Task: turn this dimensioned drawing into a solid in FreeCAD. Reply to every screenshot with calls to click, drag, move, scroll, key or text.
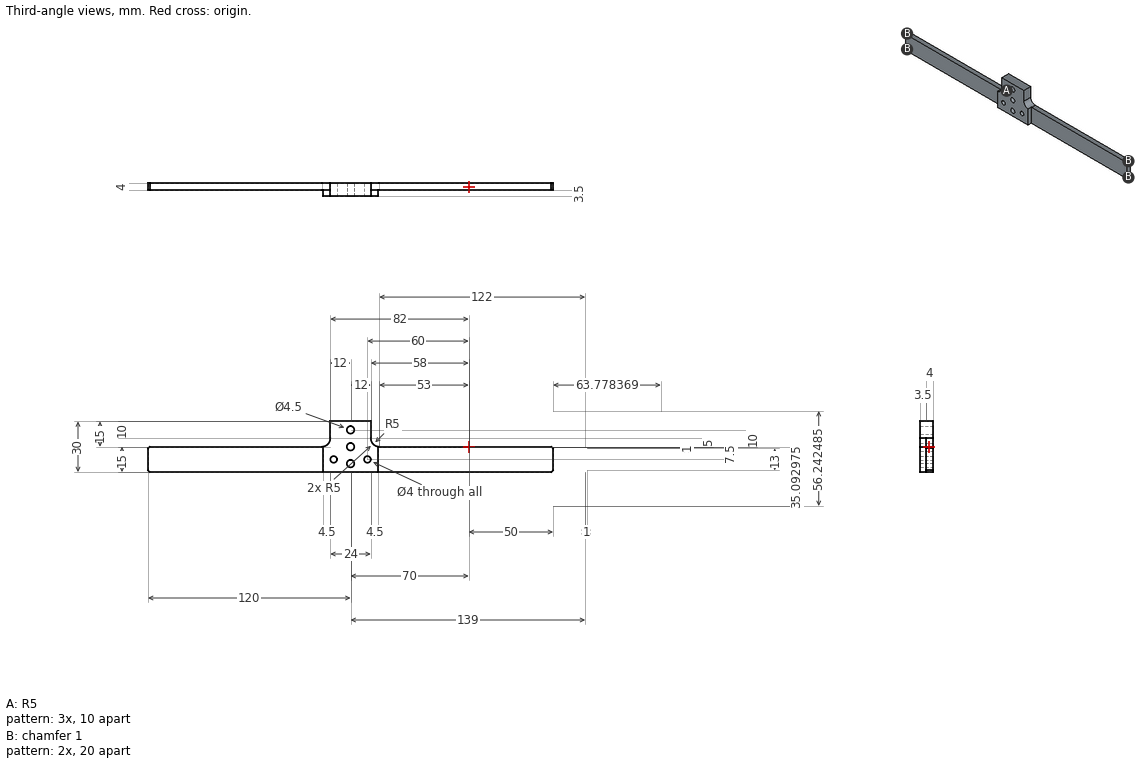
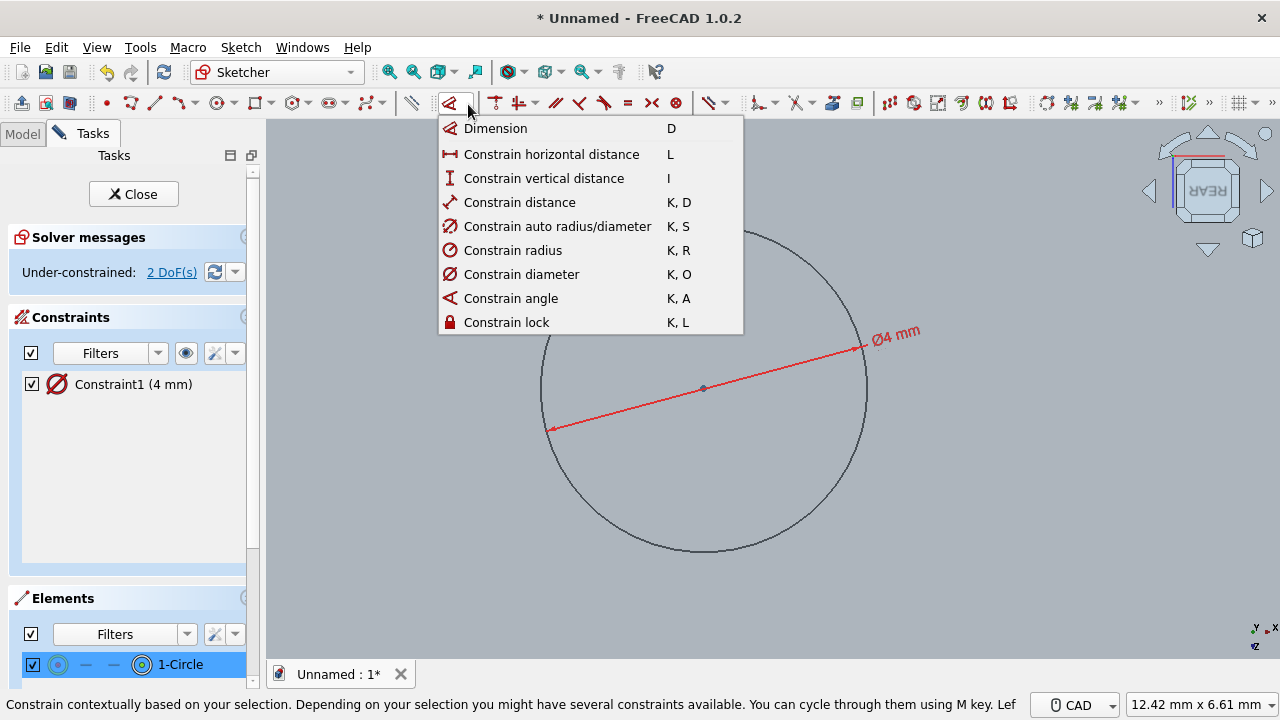
click(591, 154)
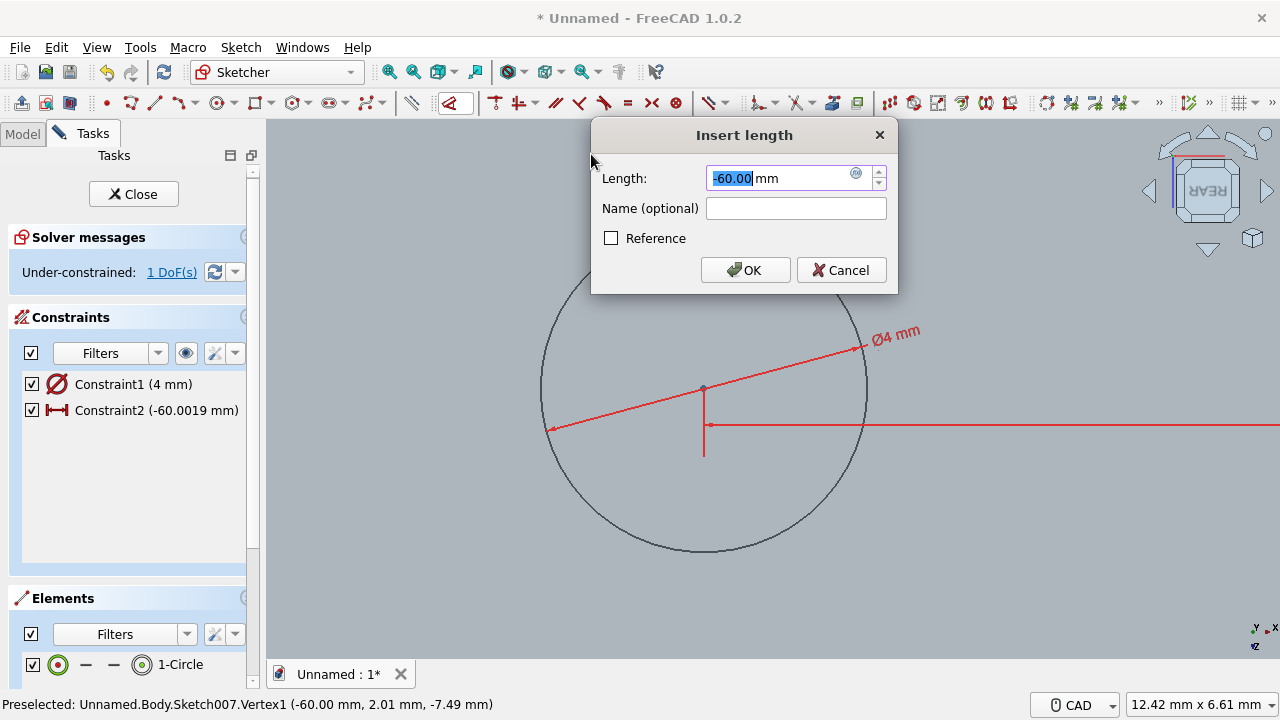
text(-60)
key(Return)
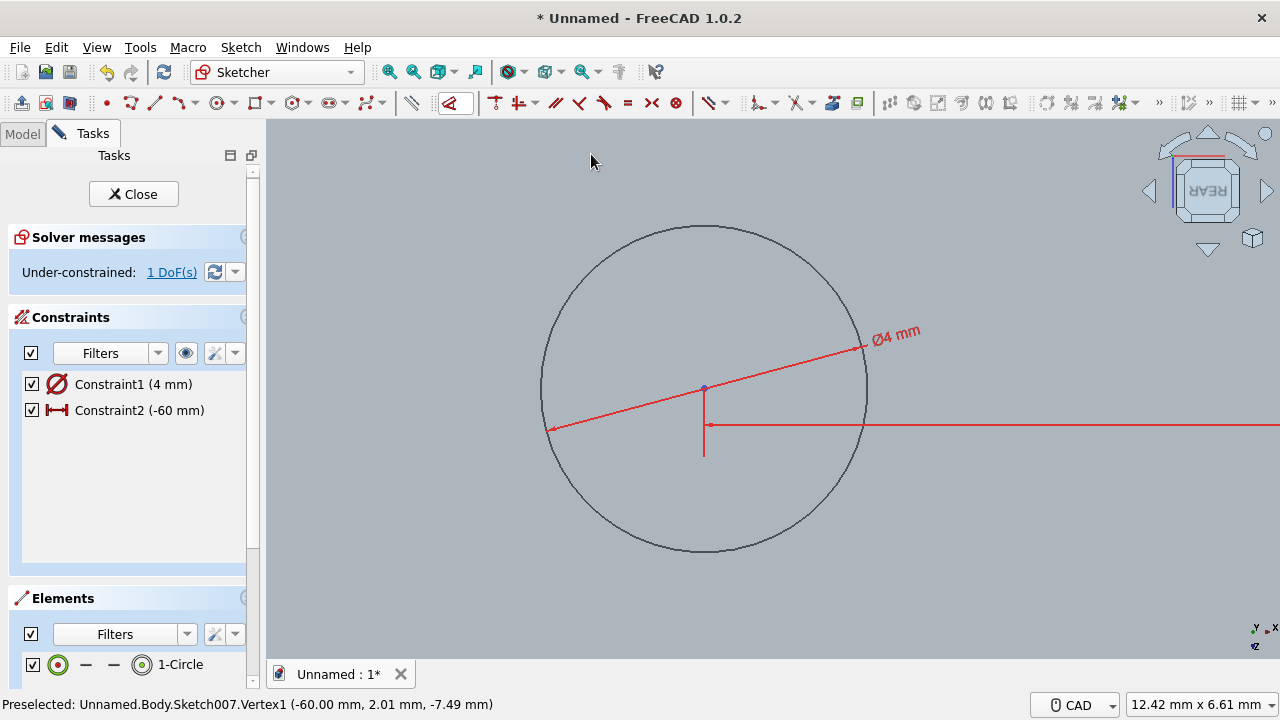
click(704, 389)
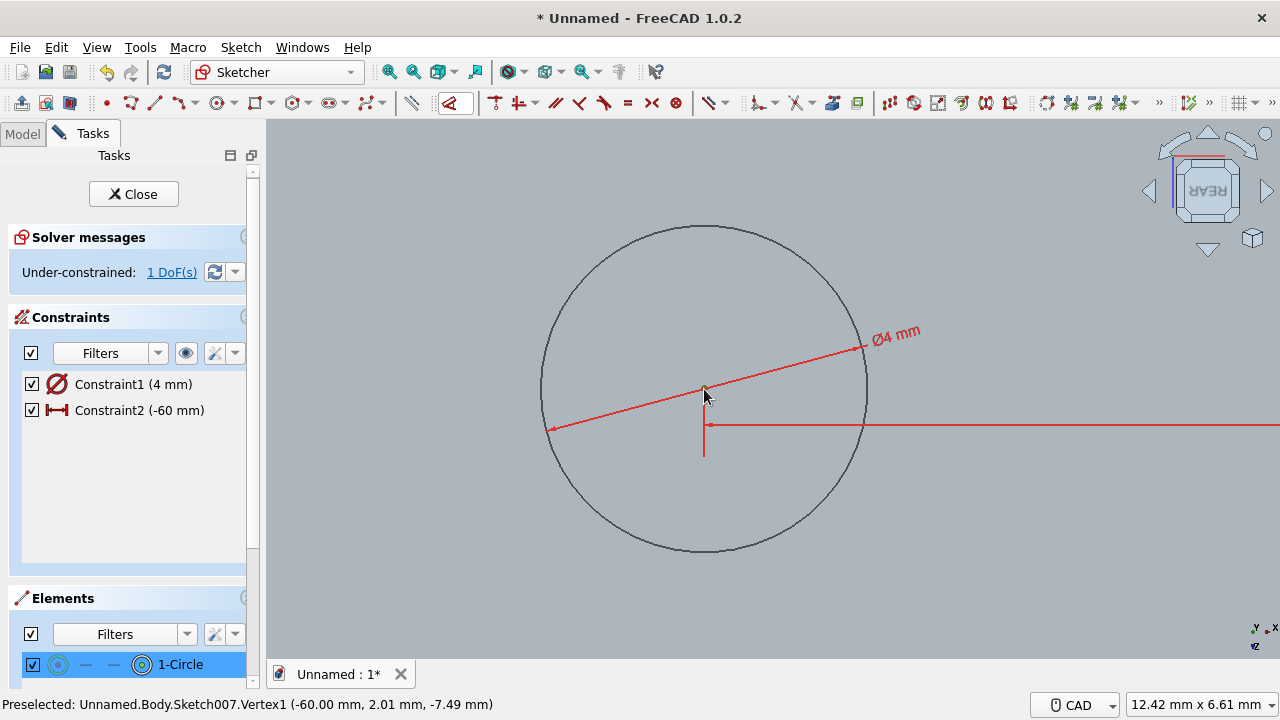
click(468, 104)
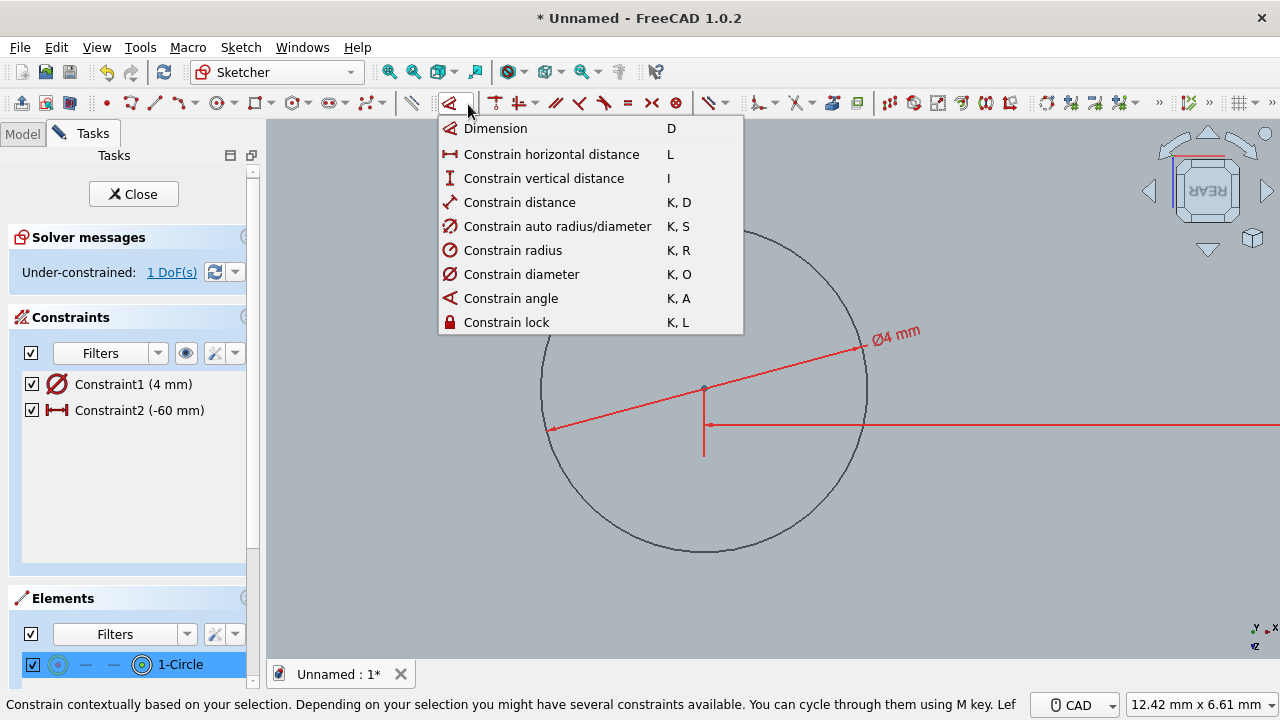
click(591, 178)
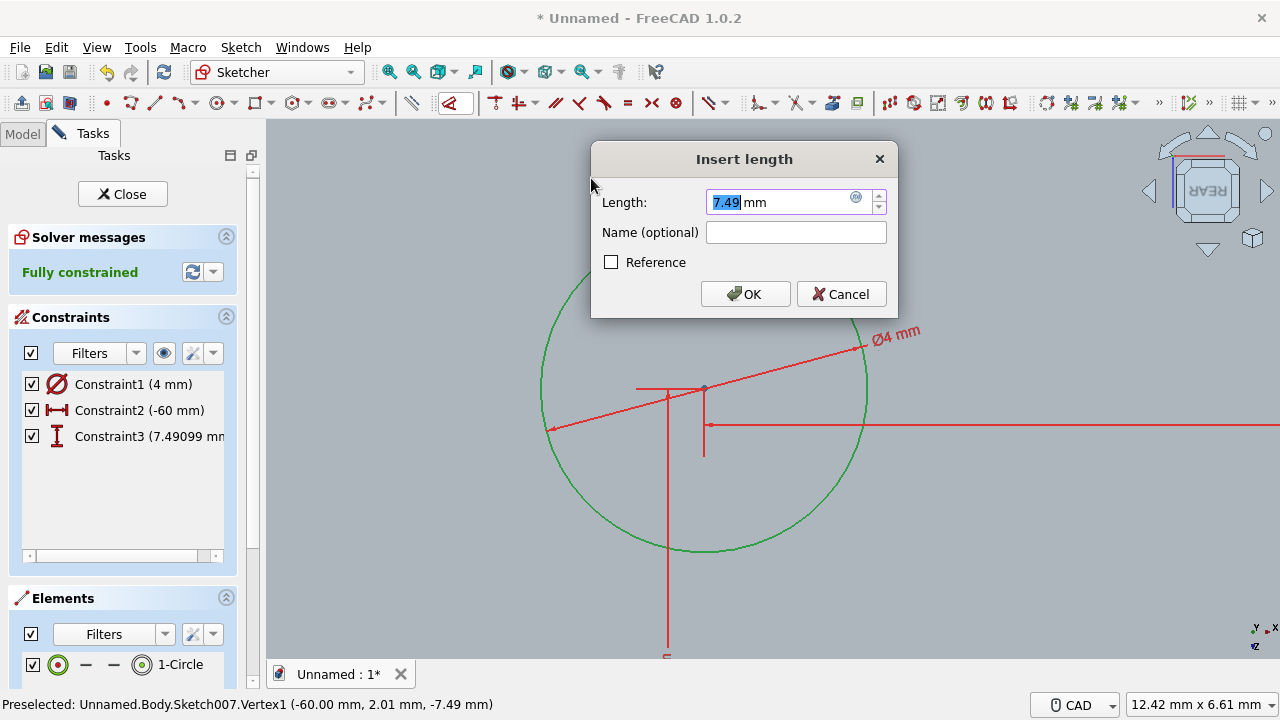
text(7.5)
key(Return)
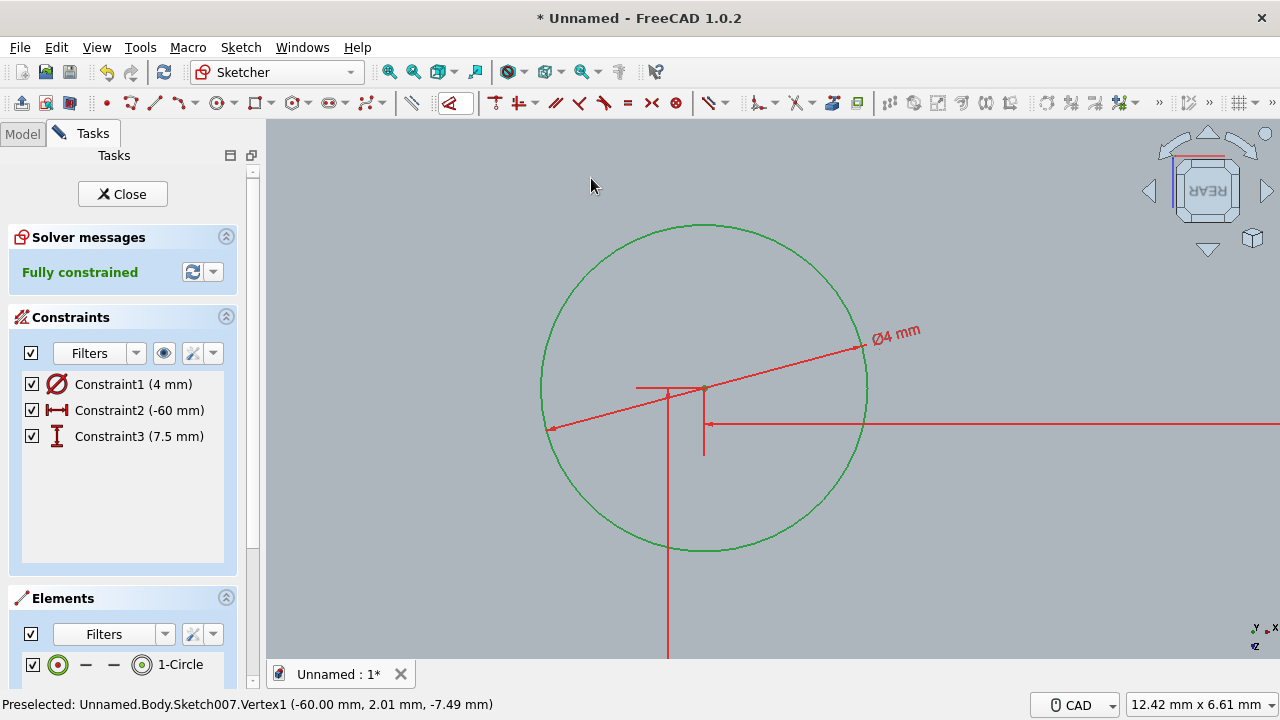
click(123, 194)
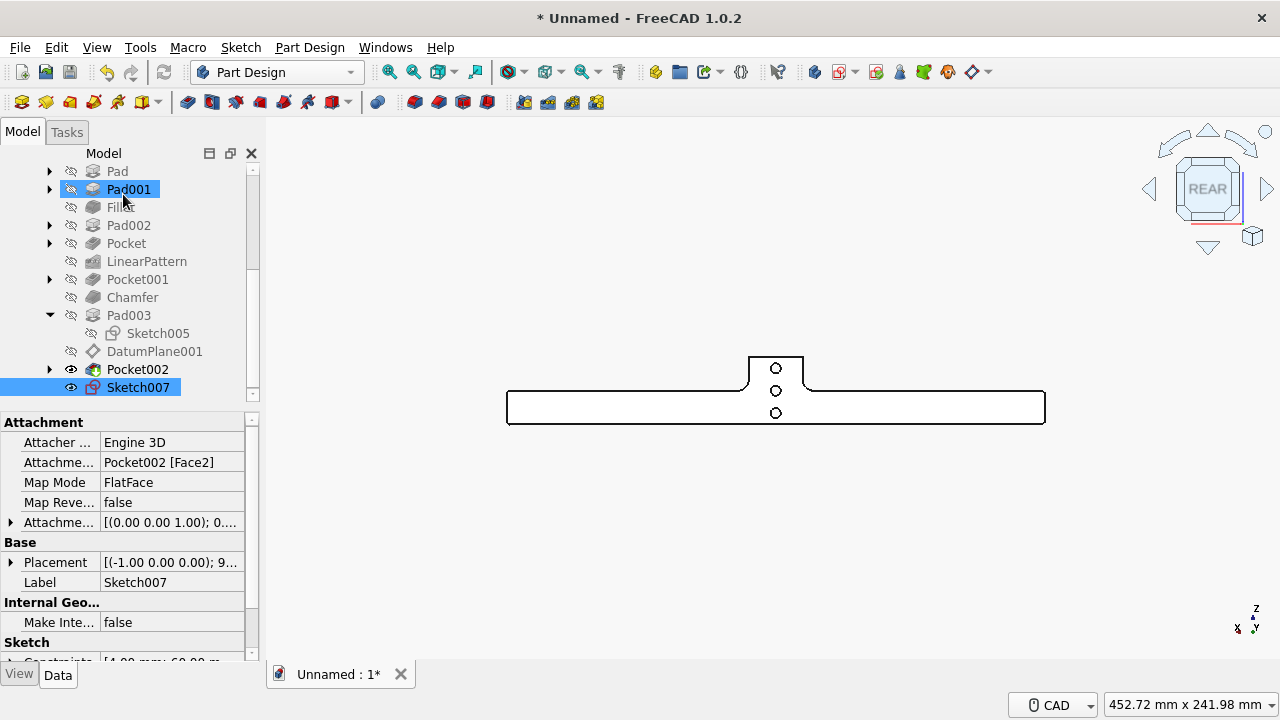
click(212, 102)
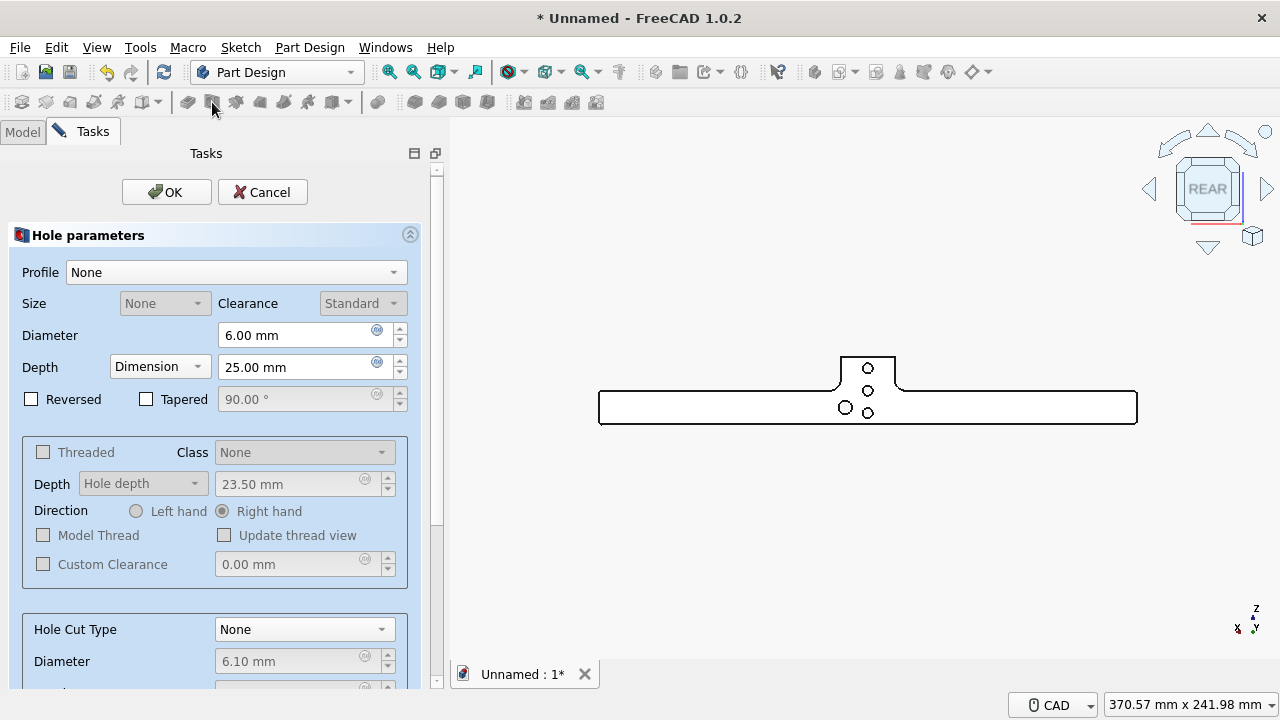
triple_click(305, 335)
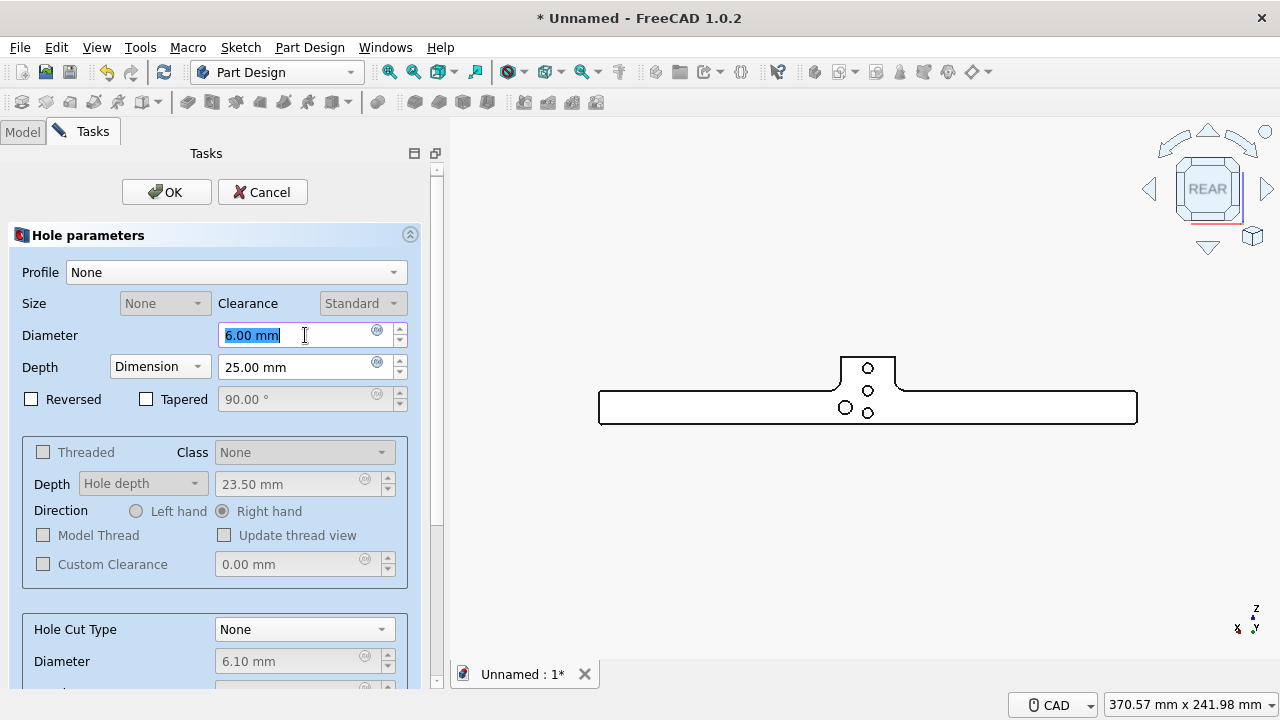
text(4)
key(Tab)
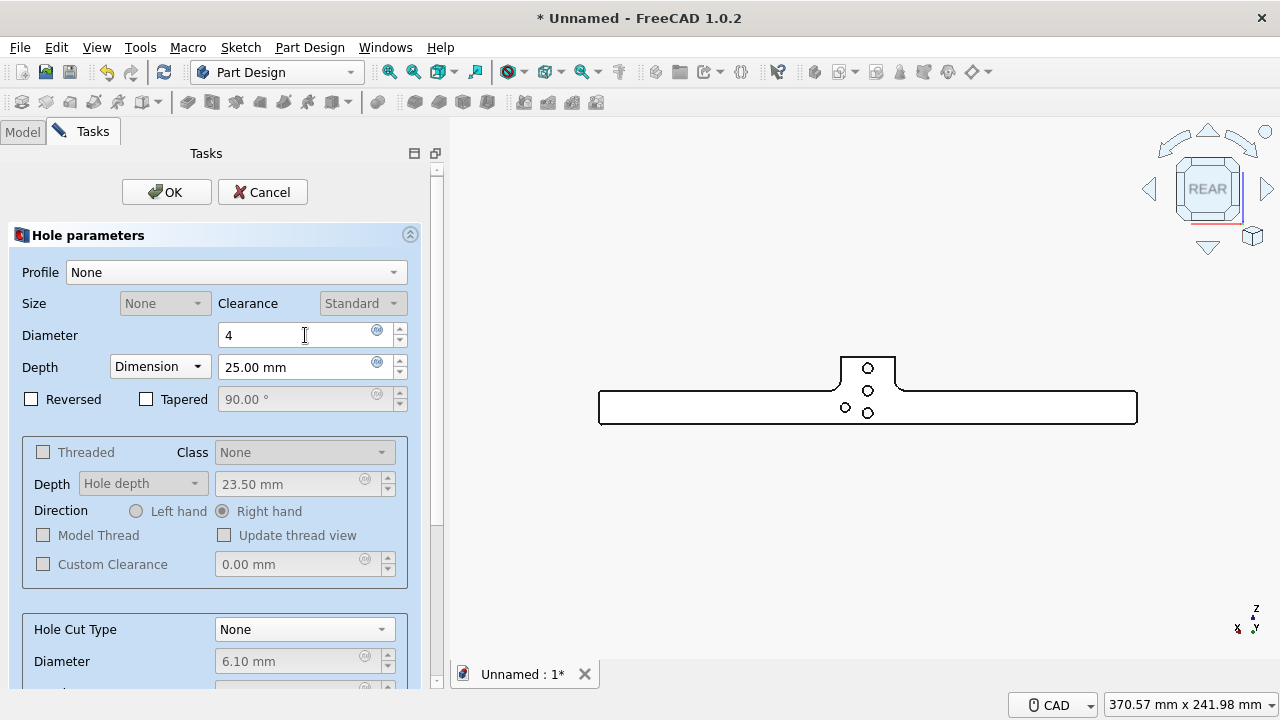
click(161, 366)